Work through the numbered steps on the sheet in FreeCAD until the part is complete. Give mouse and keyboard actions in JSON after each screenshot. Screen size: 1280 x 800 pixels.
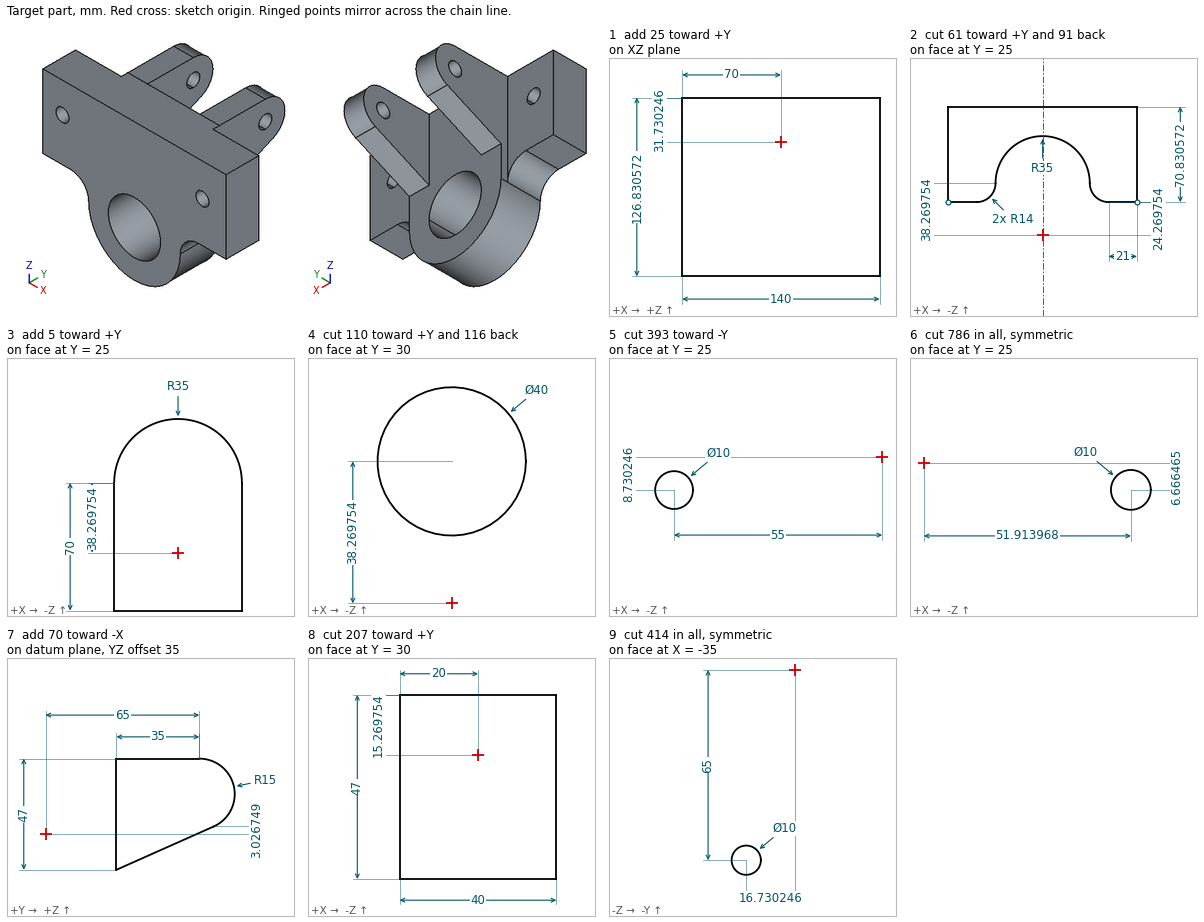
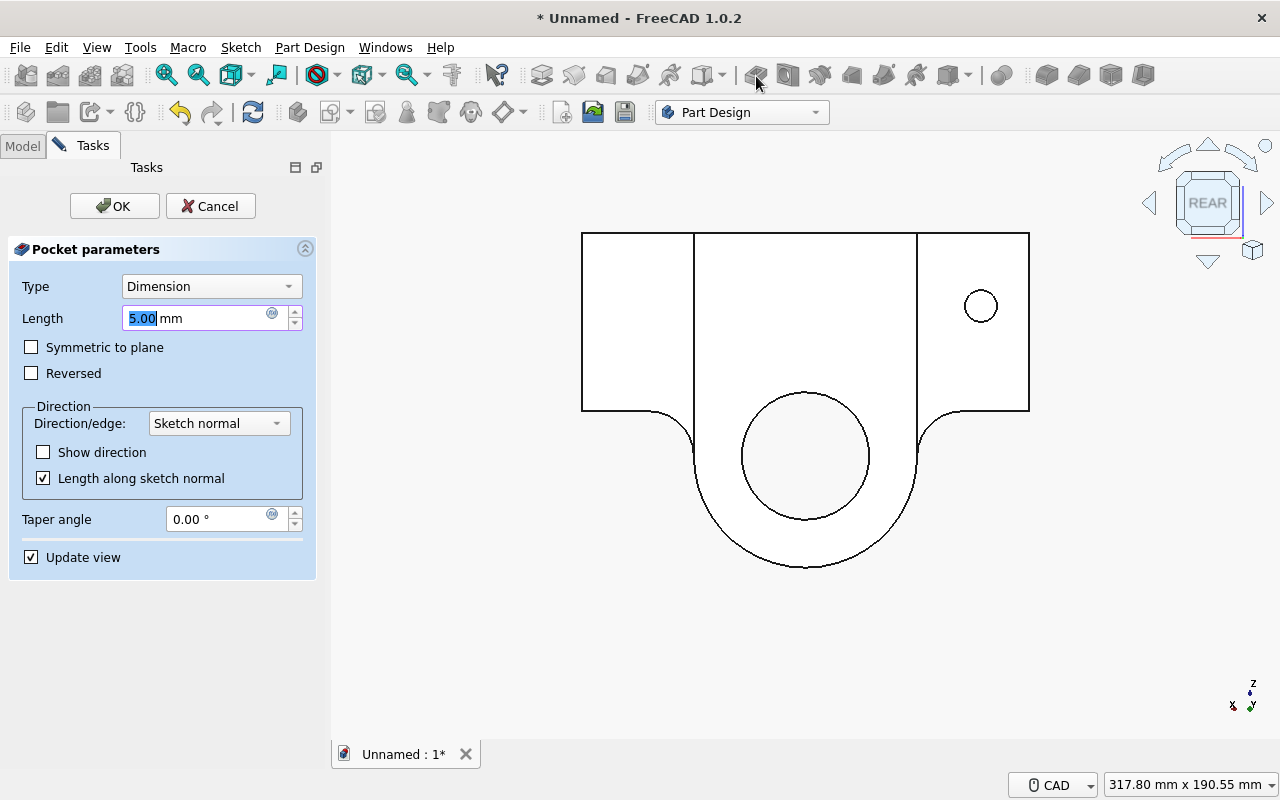
{"action": "type", "text": "393"}
{"action": "key", "text": "Tab"}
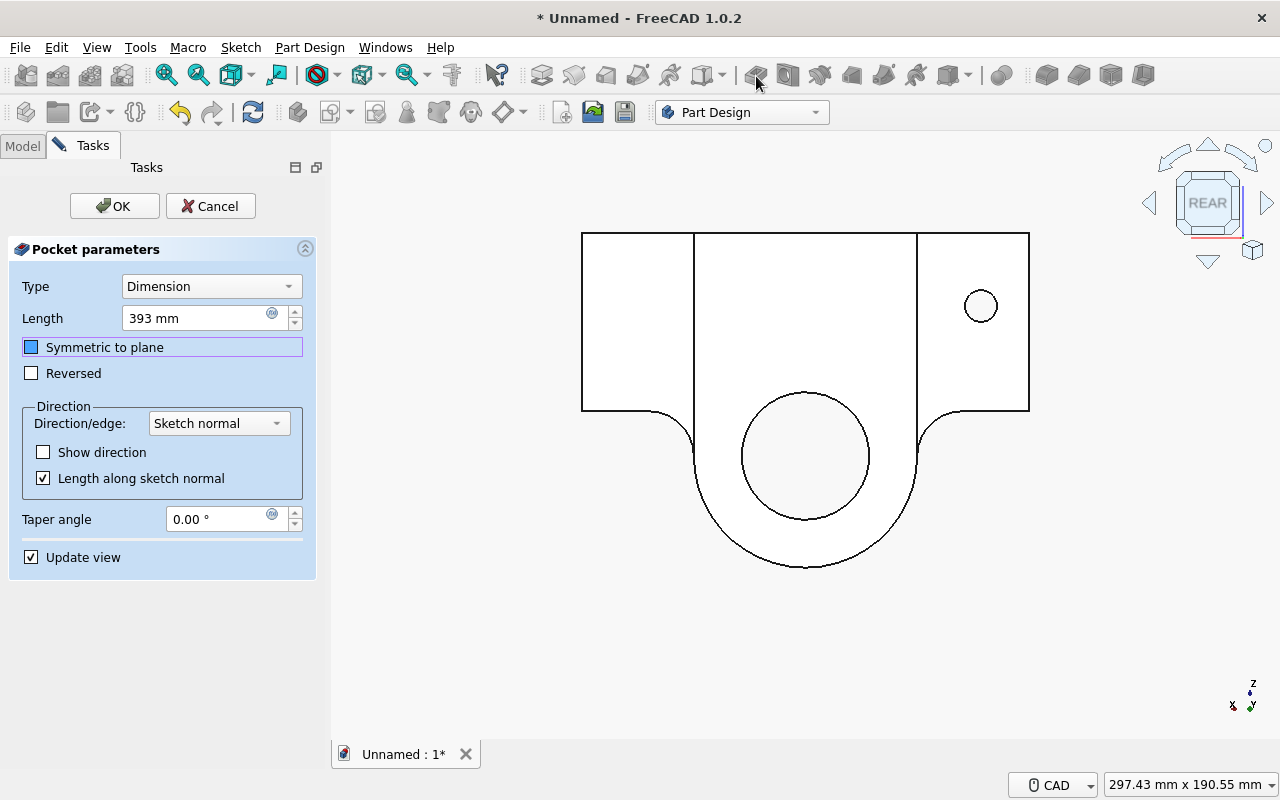
{"action": "left_click", "coordinate": [115, 206]}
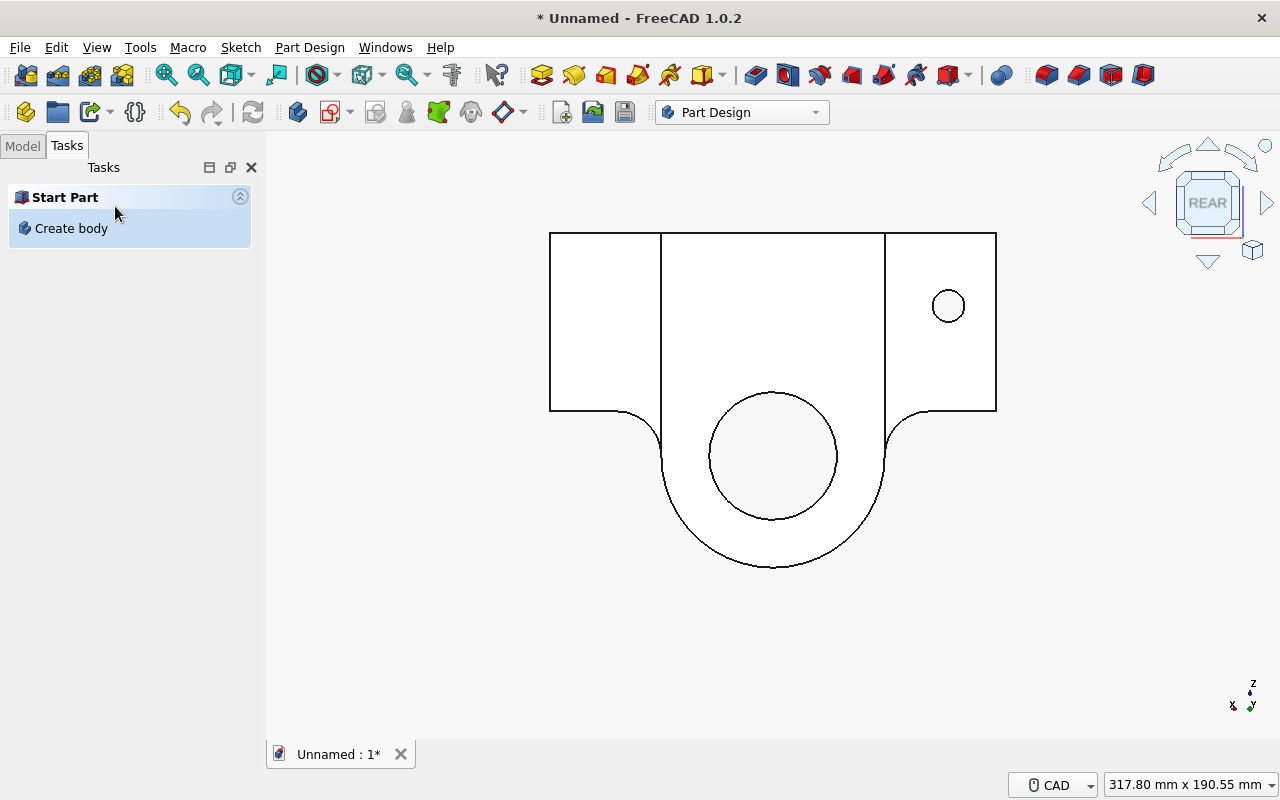
{"action": "left_click", "coordinate": [605, 311]}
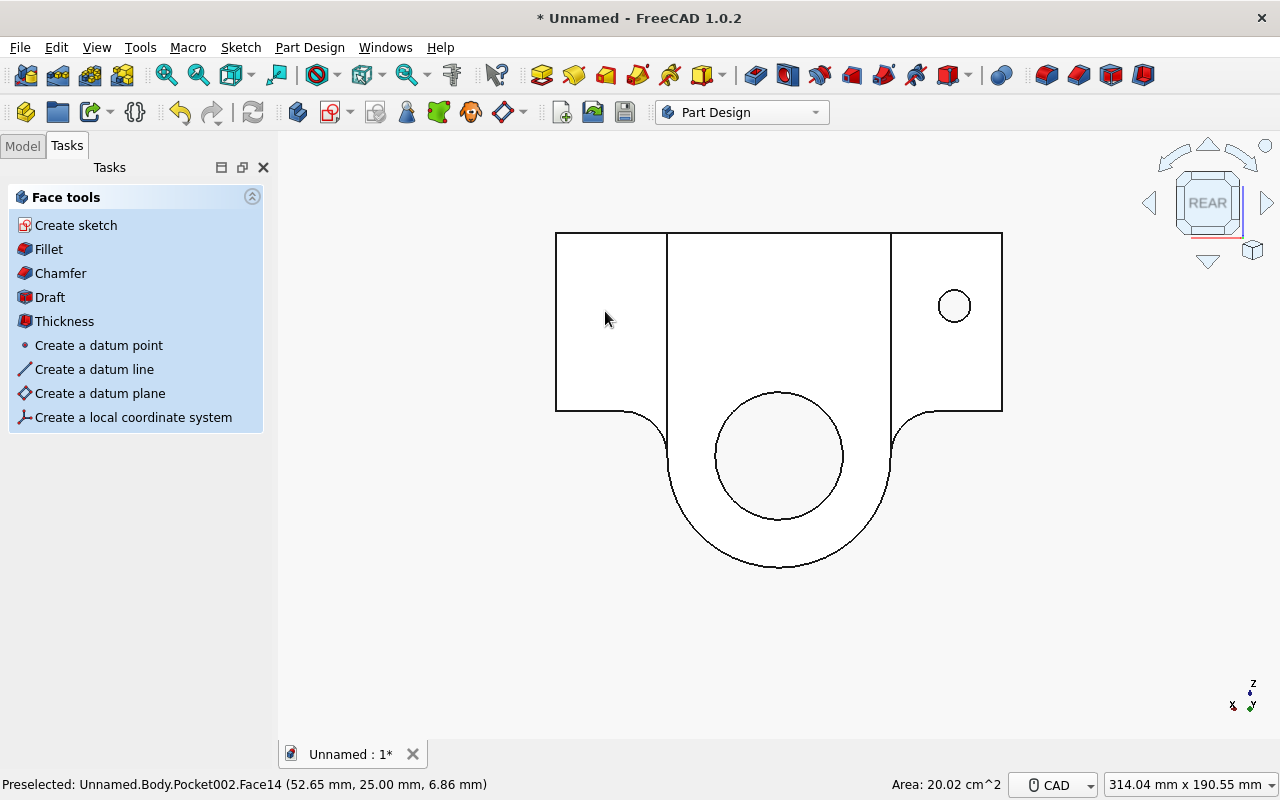
{"action": "left_click", "coordinate": [330, 112]}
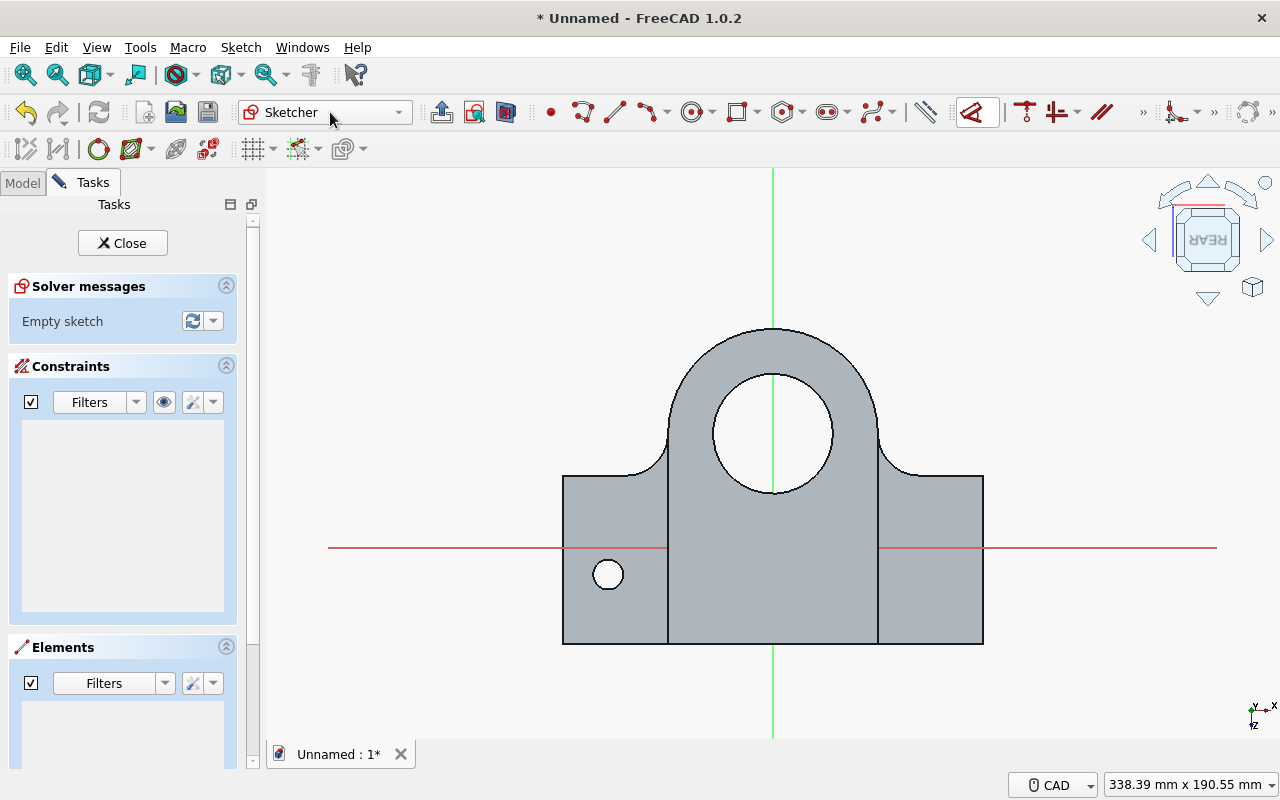
{"action": "scroll", "coordinate": [951, 580], "scroll_direction": "up", "scroll_amount": 12}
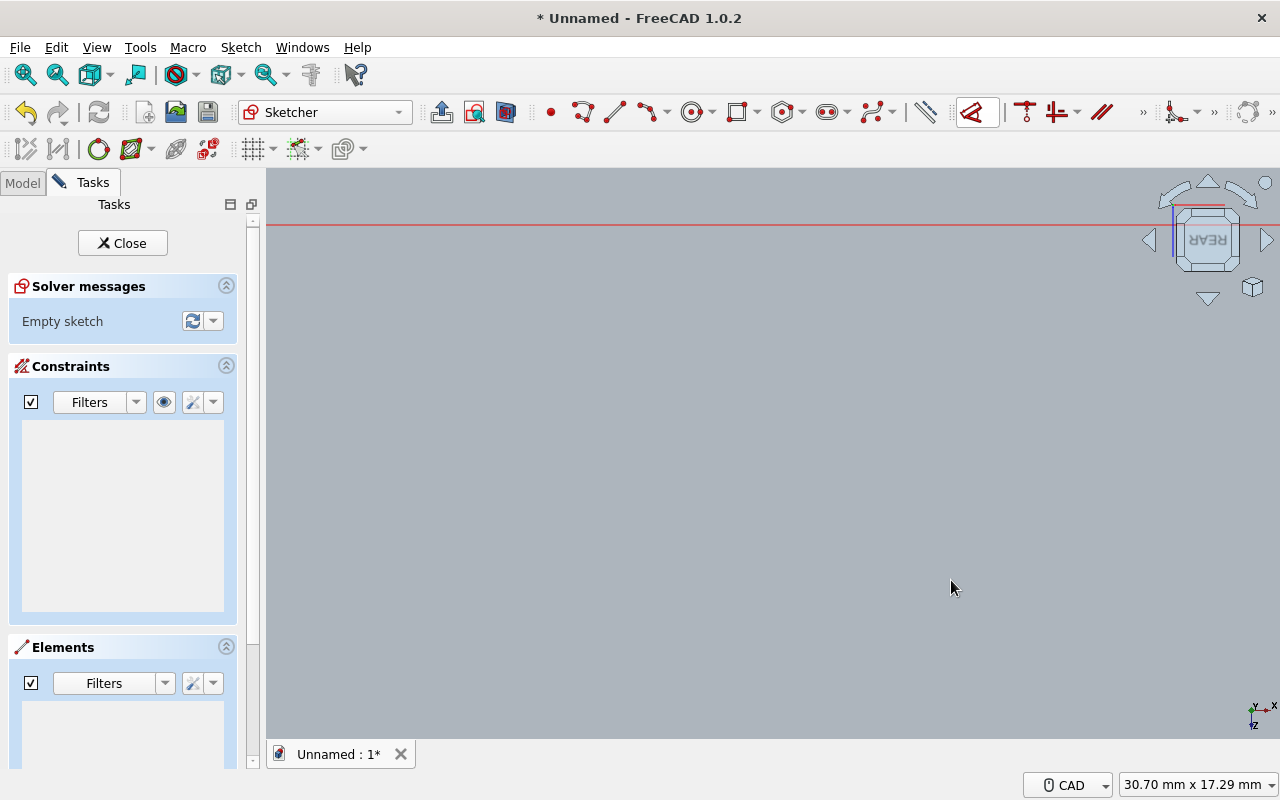
{"action": "left_click", "coordinate": [692, 112]}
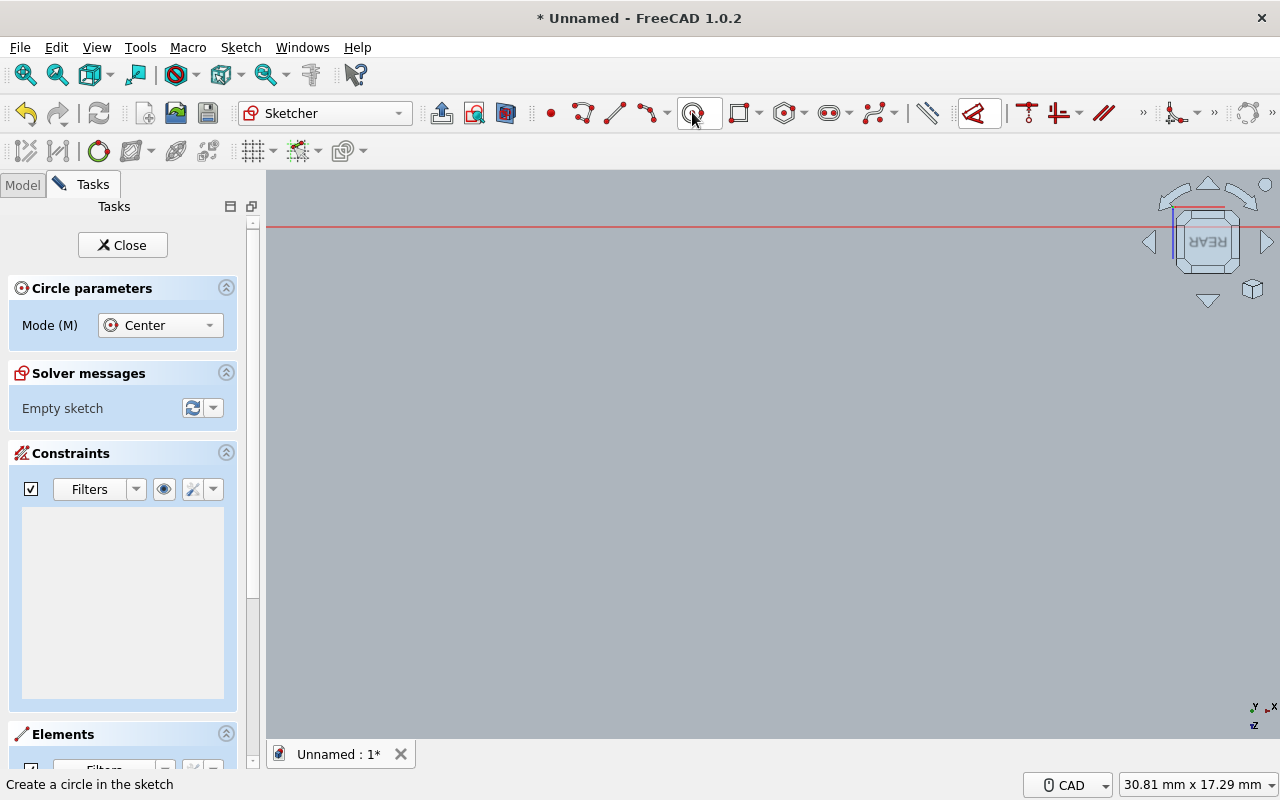
{"action": "left_click", "coordinate": [697, 446]}
{"action": "left_click", "coordinate": [814, 330]}
{"action": "key", "text": "Escape"}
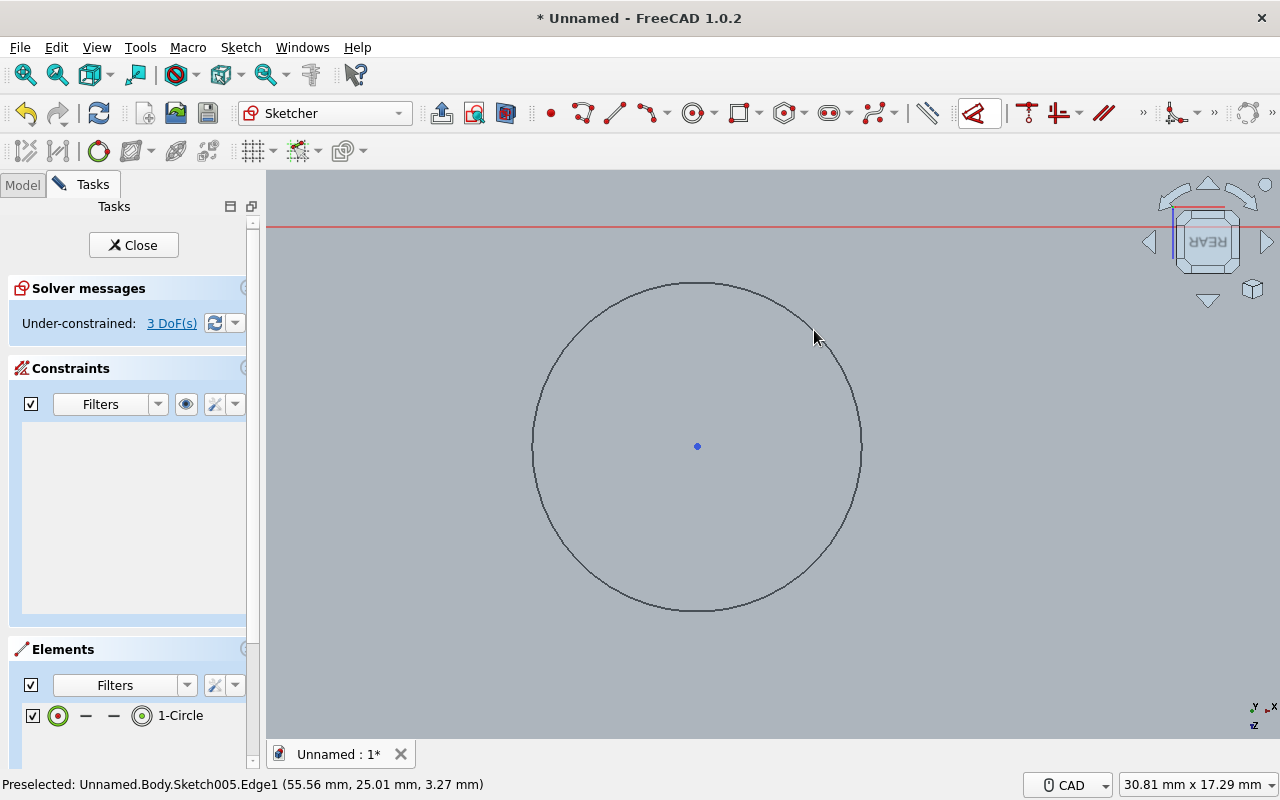
{"action": "left_click", "coordinate": [813, 330]}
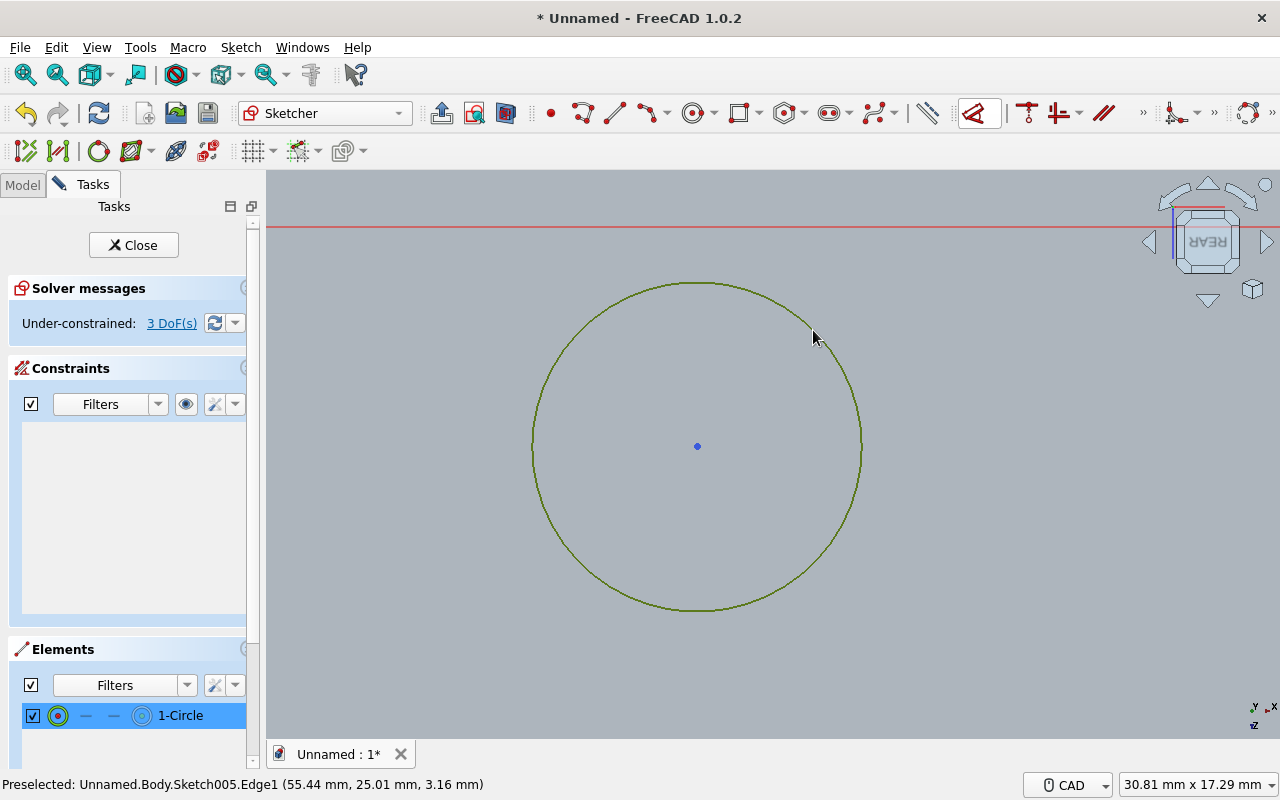
{"action": "left_click", "coordinate": [996, 114]}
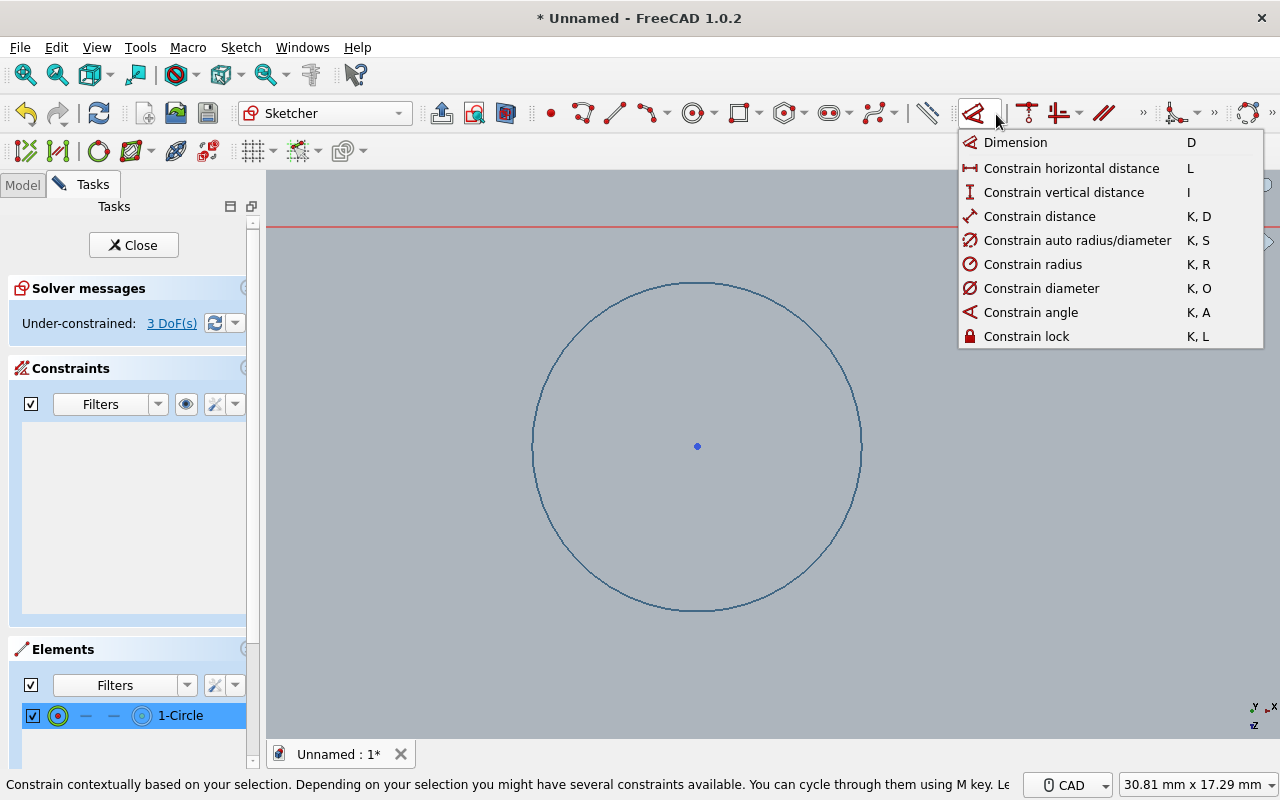
{"action": "left_click", "coordinate": [1111, 288]}